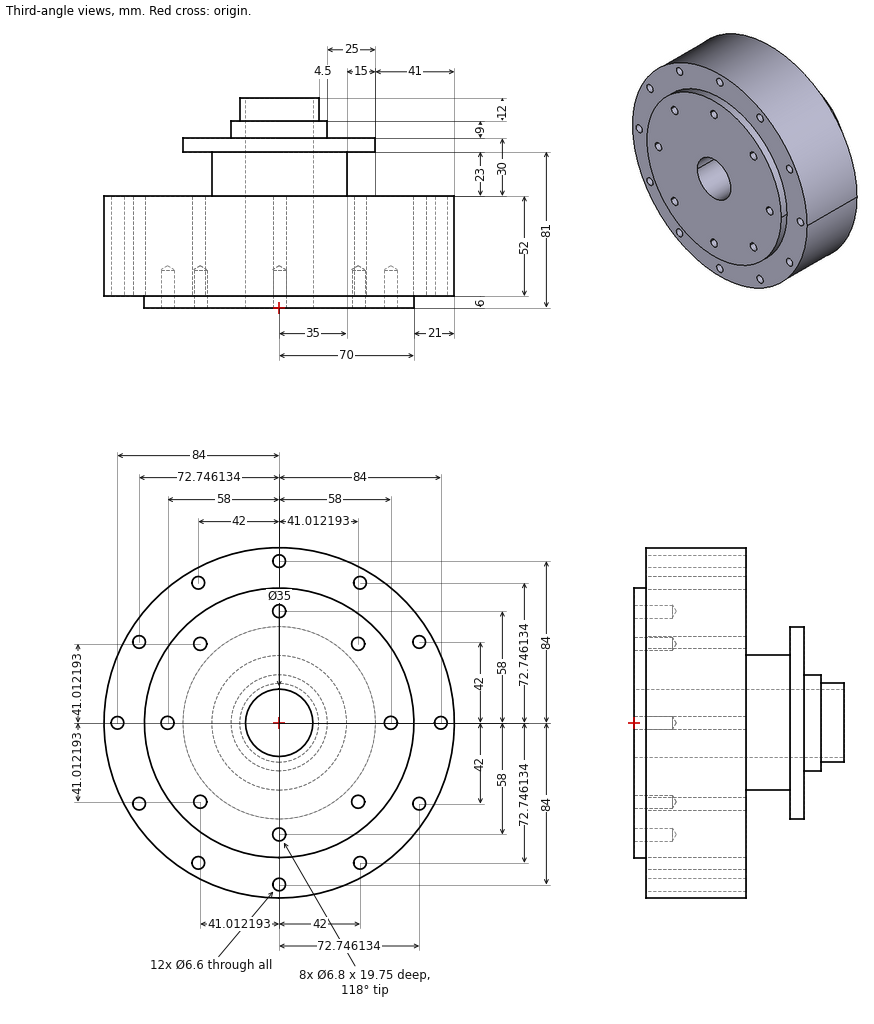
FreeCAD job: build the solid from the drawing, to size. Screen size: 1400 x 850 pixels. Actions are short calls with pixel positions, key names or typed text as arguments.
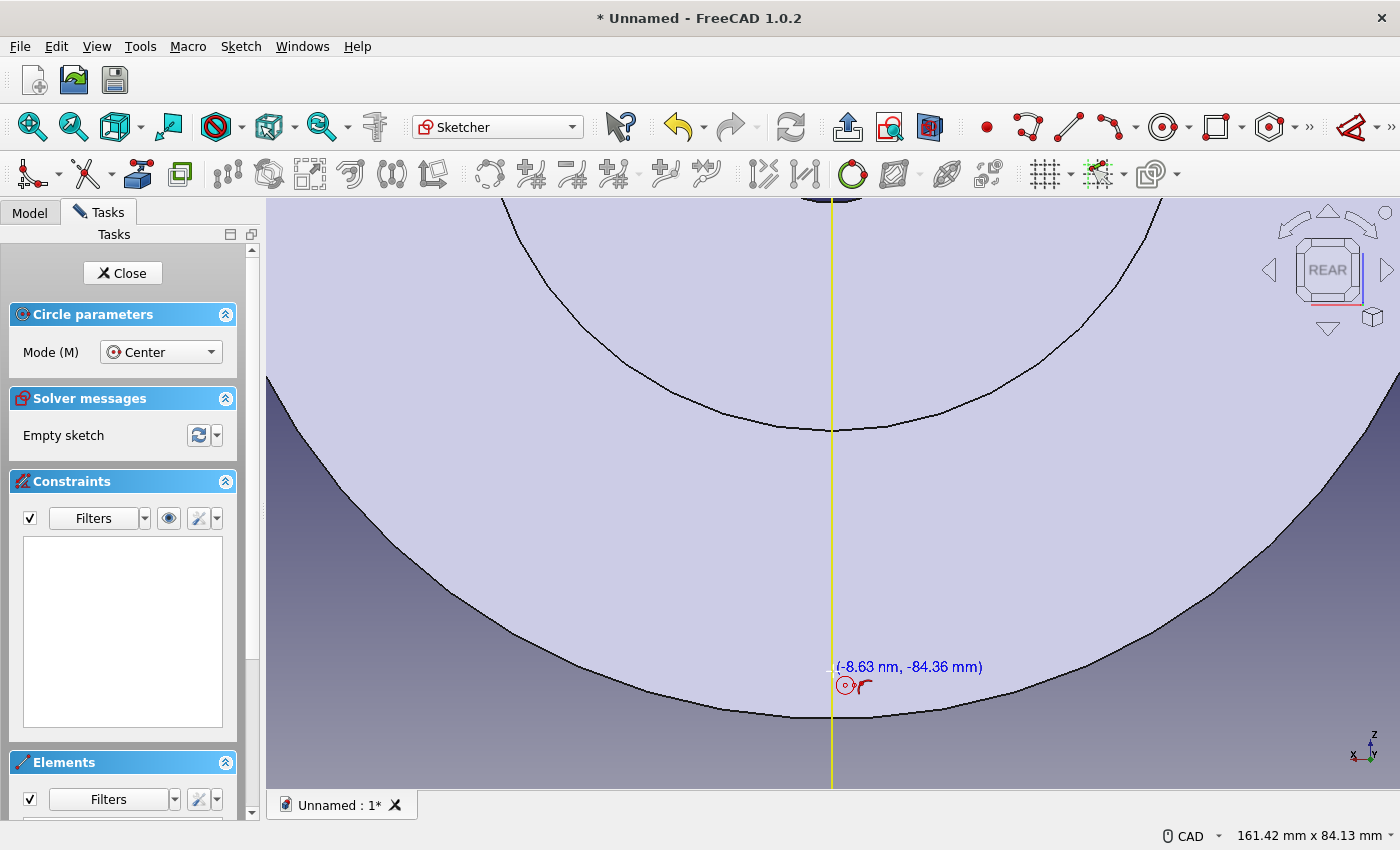
click(832, 670)
click(848, 654)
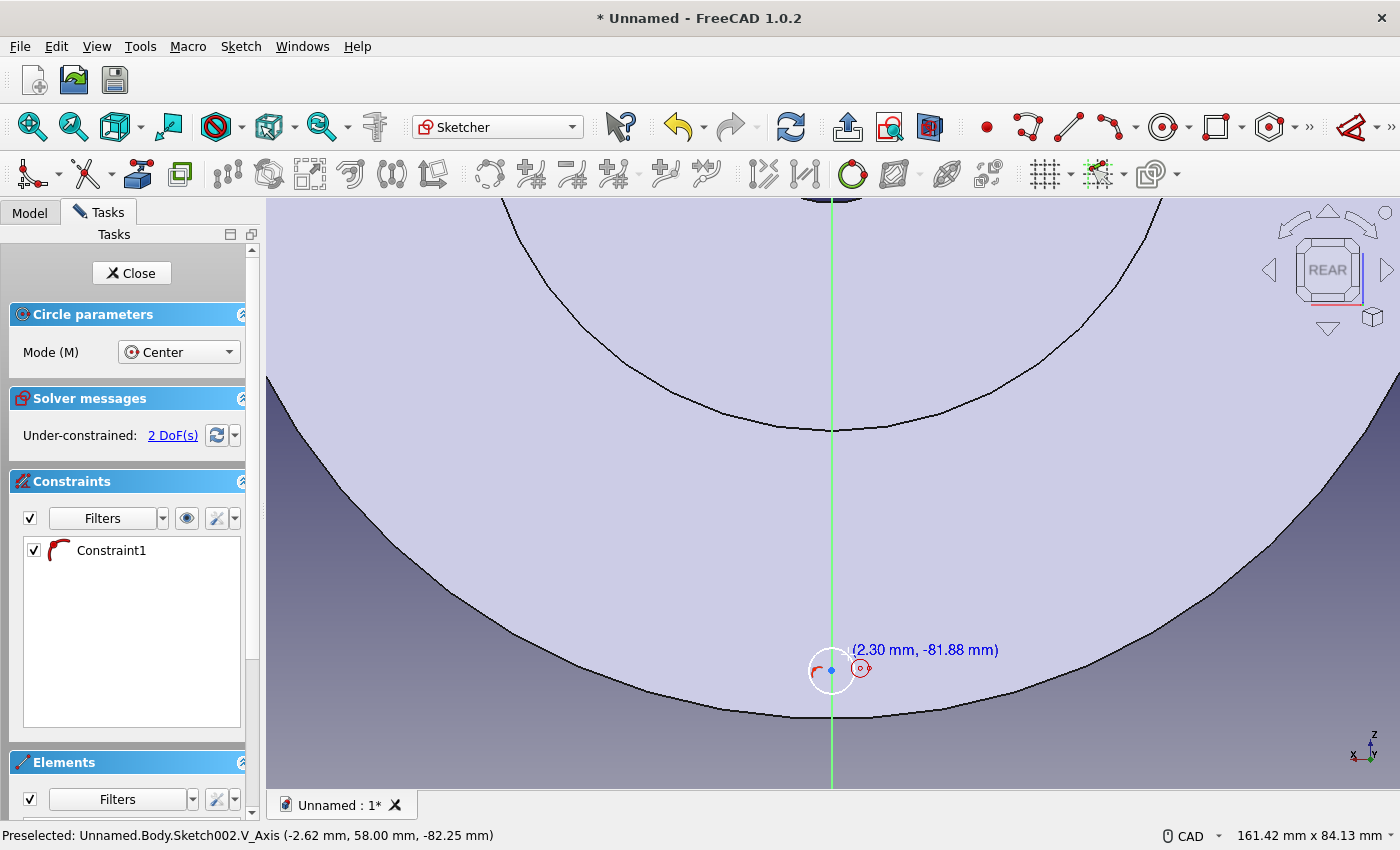
click(537, 591)
click(553, 574)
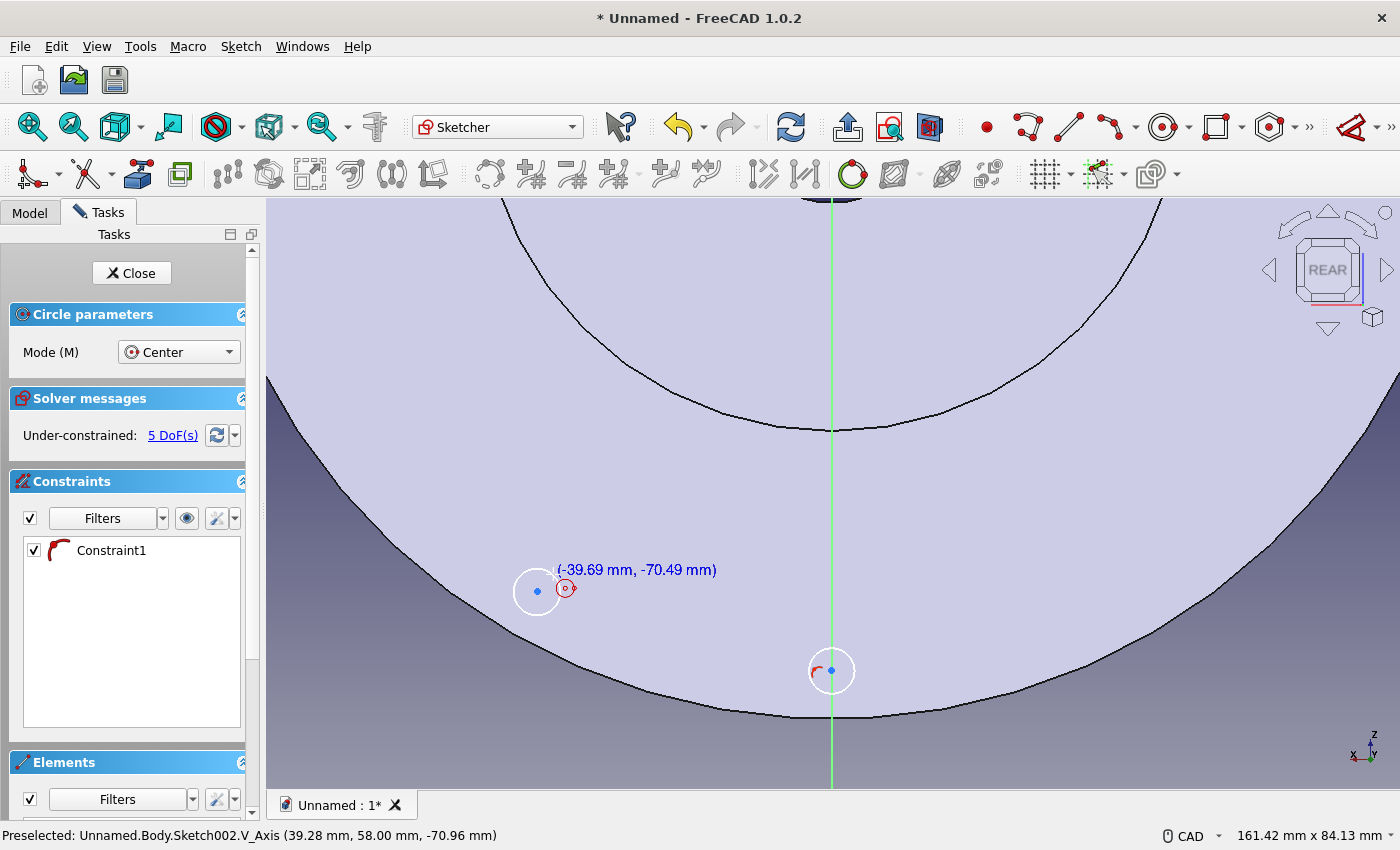
click(321, 375)
click(337, 358)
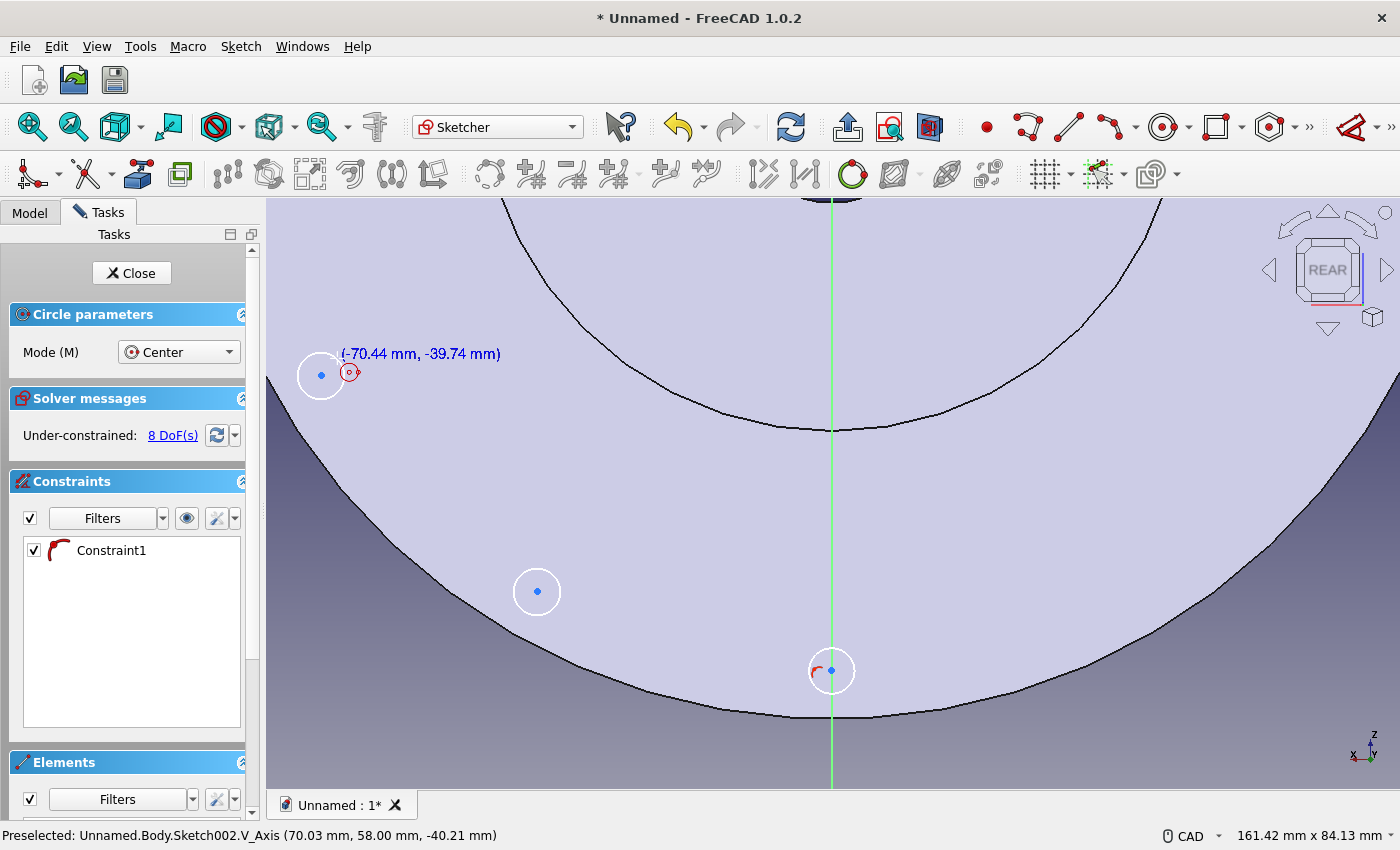
scroll(735, 672, down, 6)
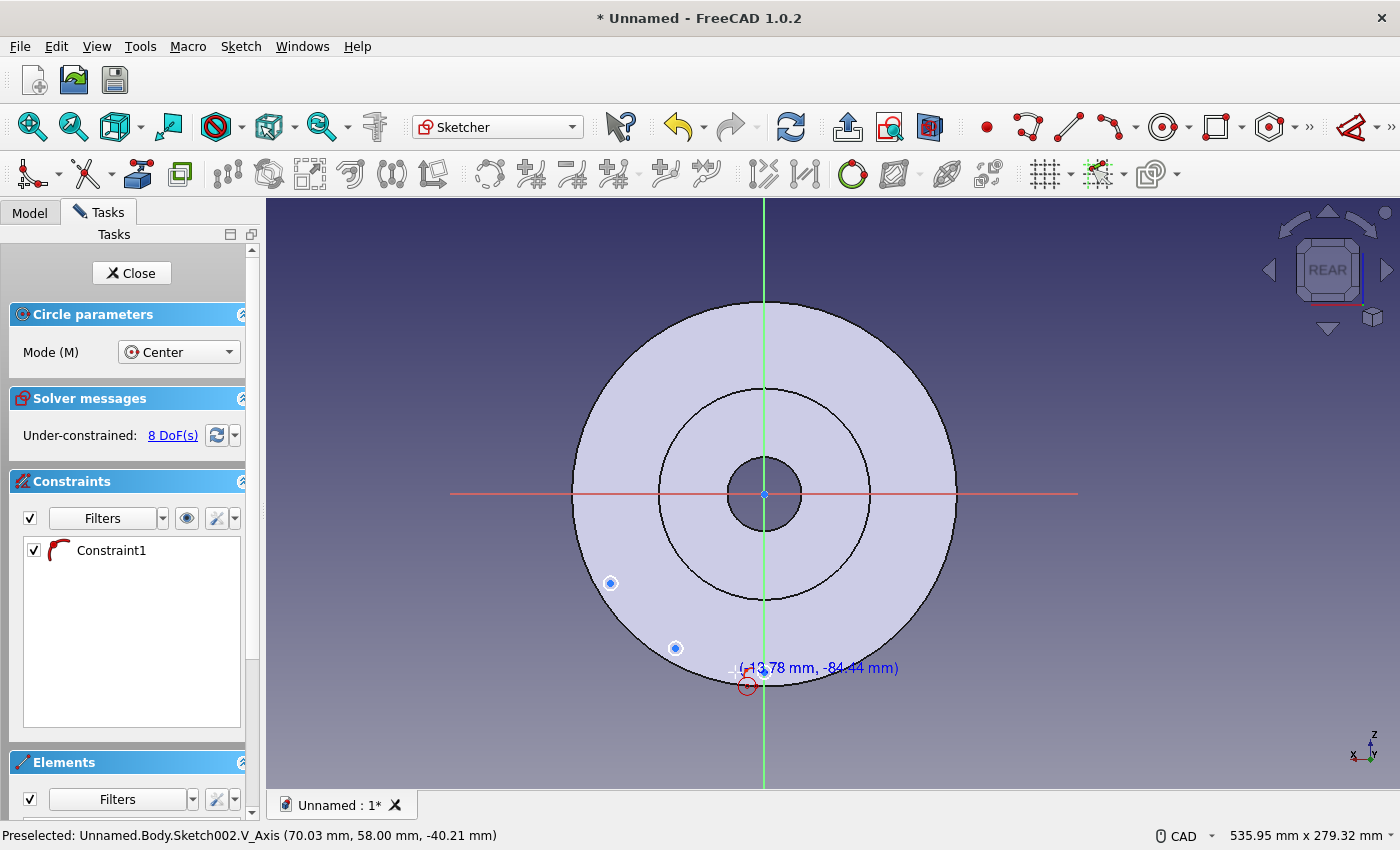
scroll(587, 494, up, 6)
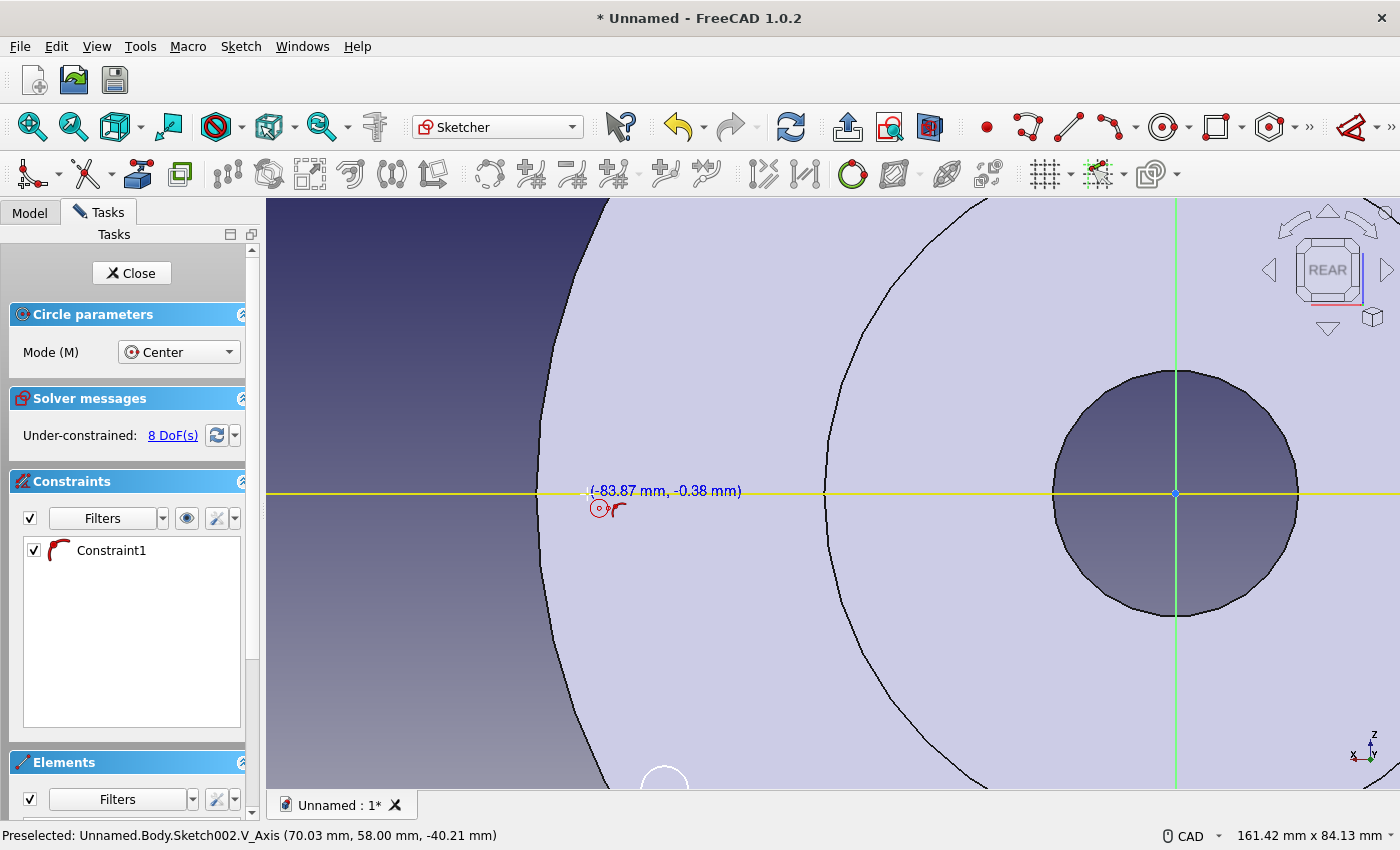
click(585, 494)
click(602, 477)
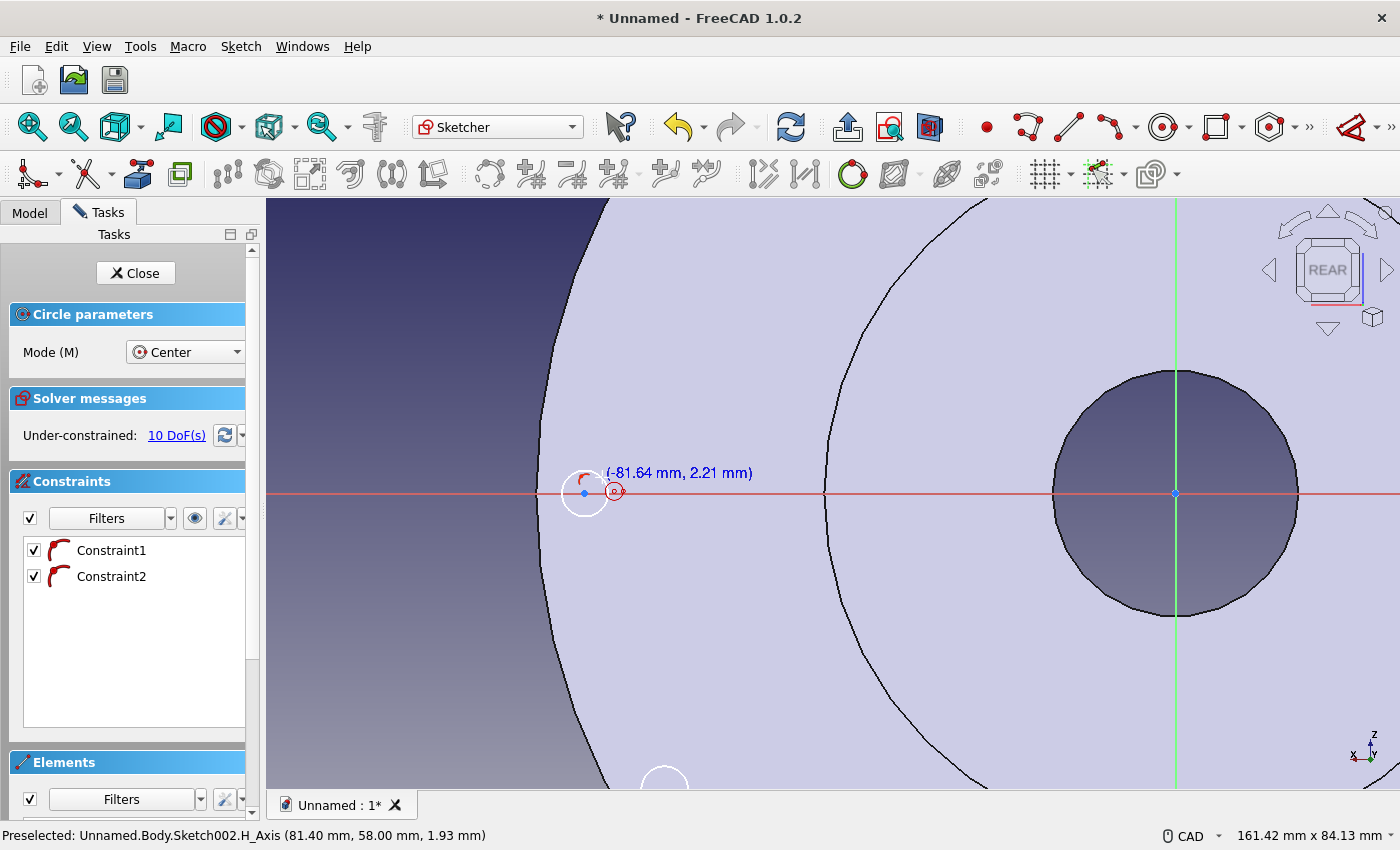
scroll(587, 493, down, 6)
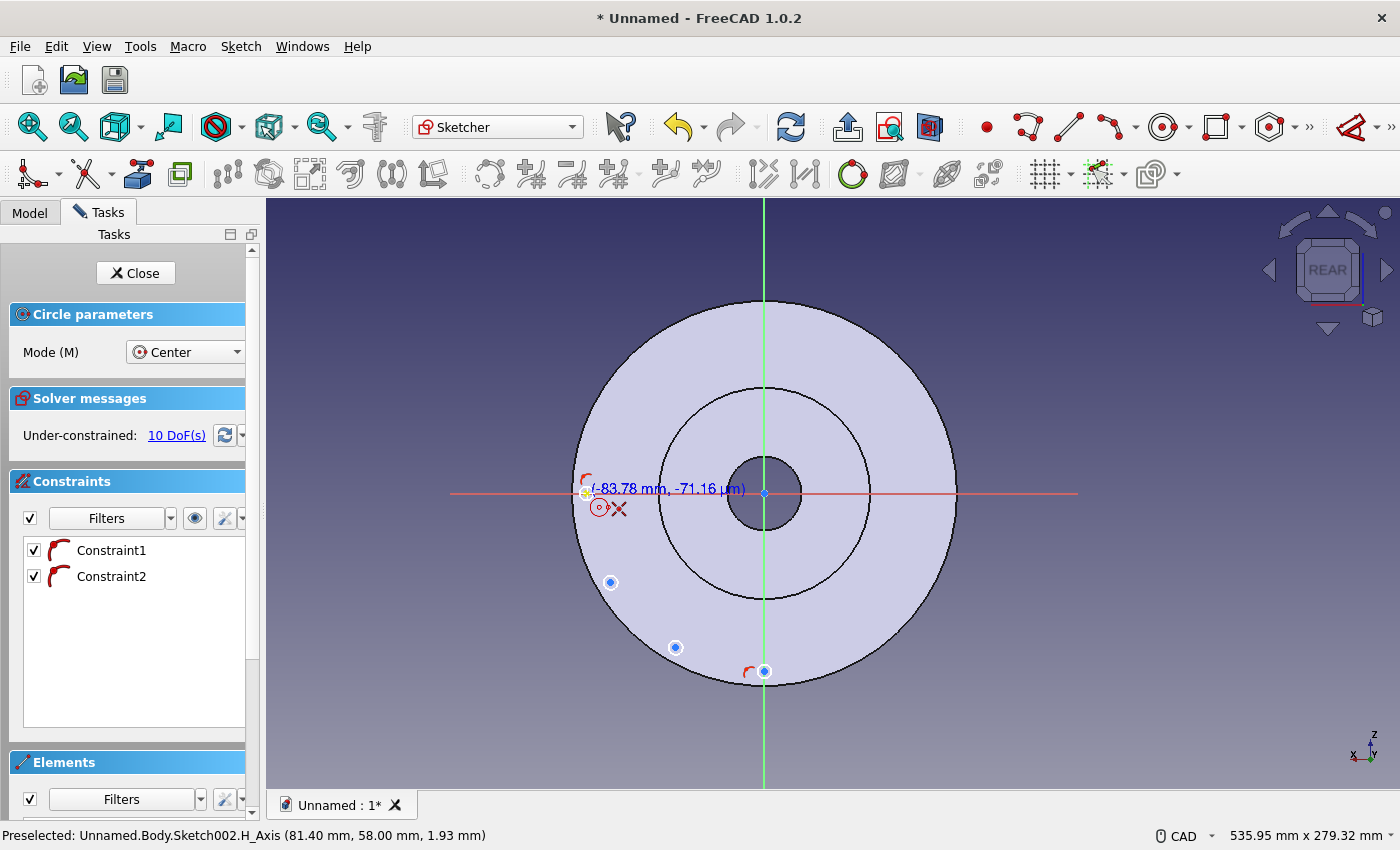
scroll(611, 405, up, 6)